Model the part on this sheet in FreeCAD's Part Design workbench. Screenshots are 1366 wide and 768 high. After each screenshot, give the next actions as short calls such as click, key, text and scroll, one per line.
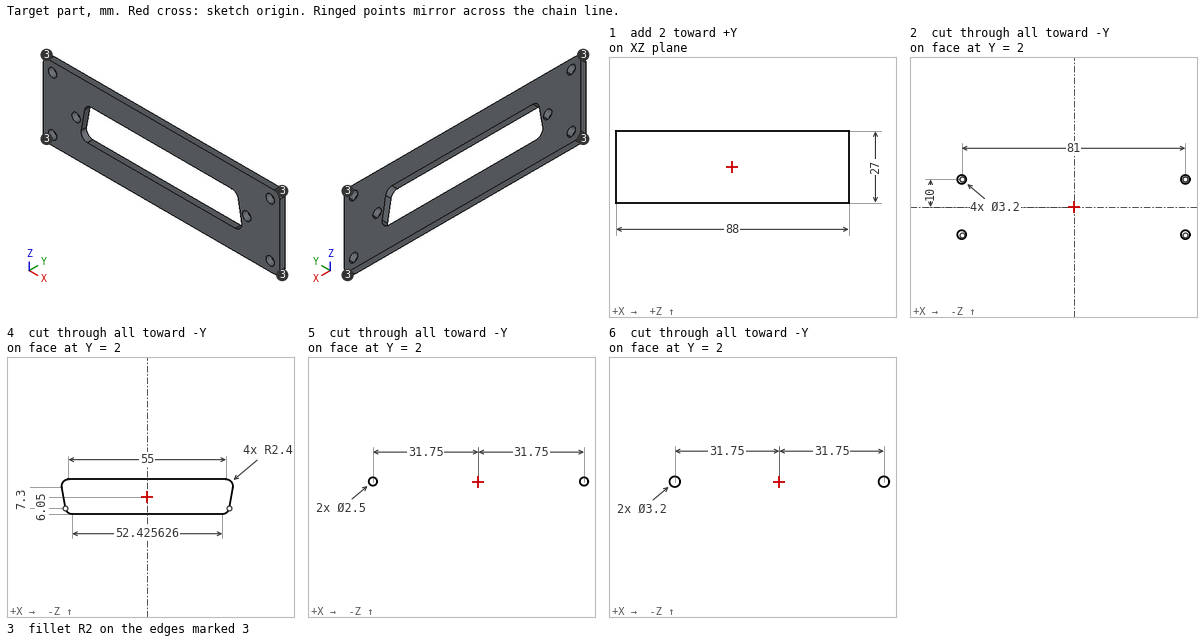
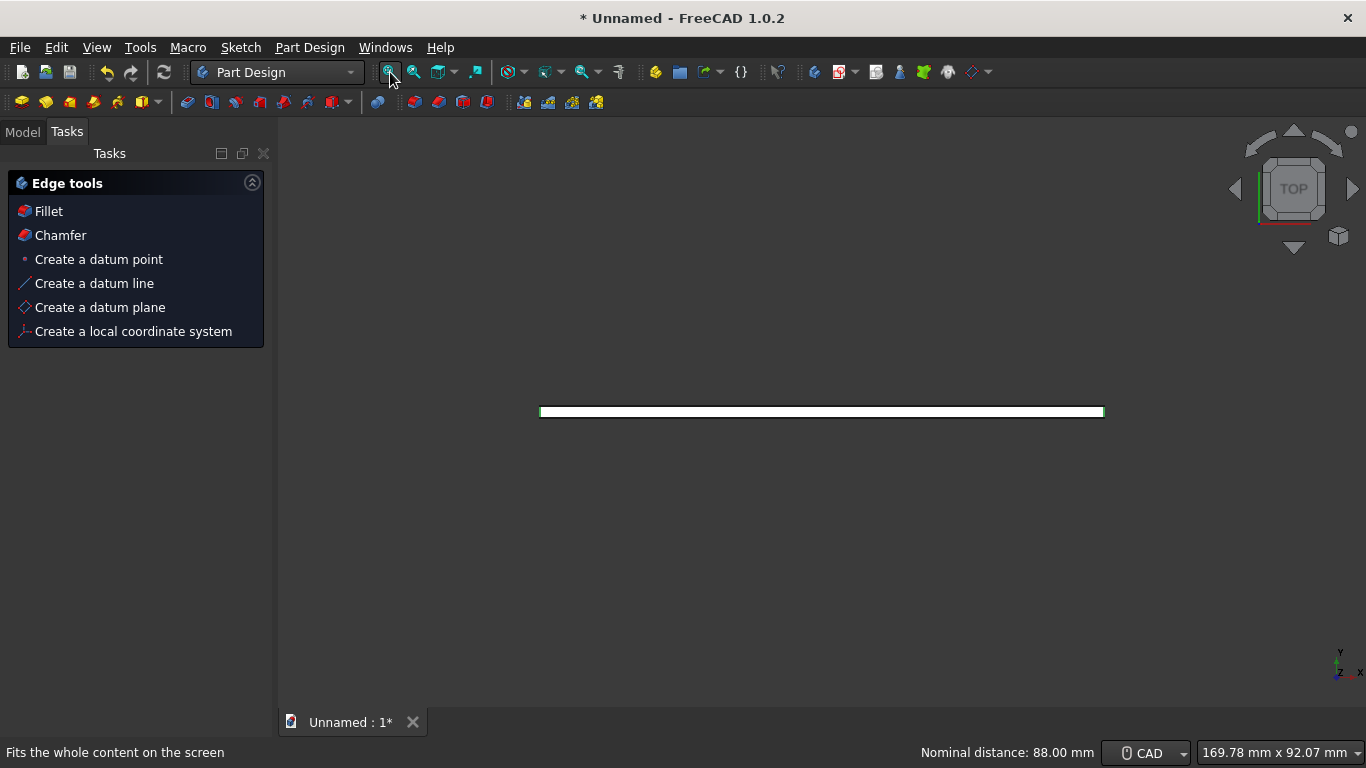
key(1)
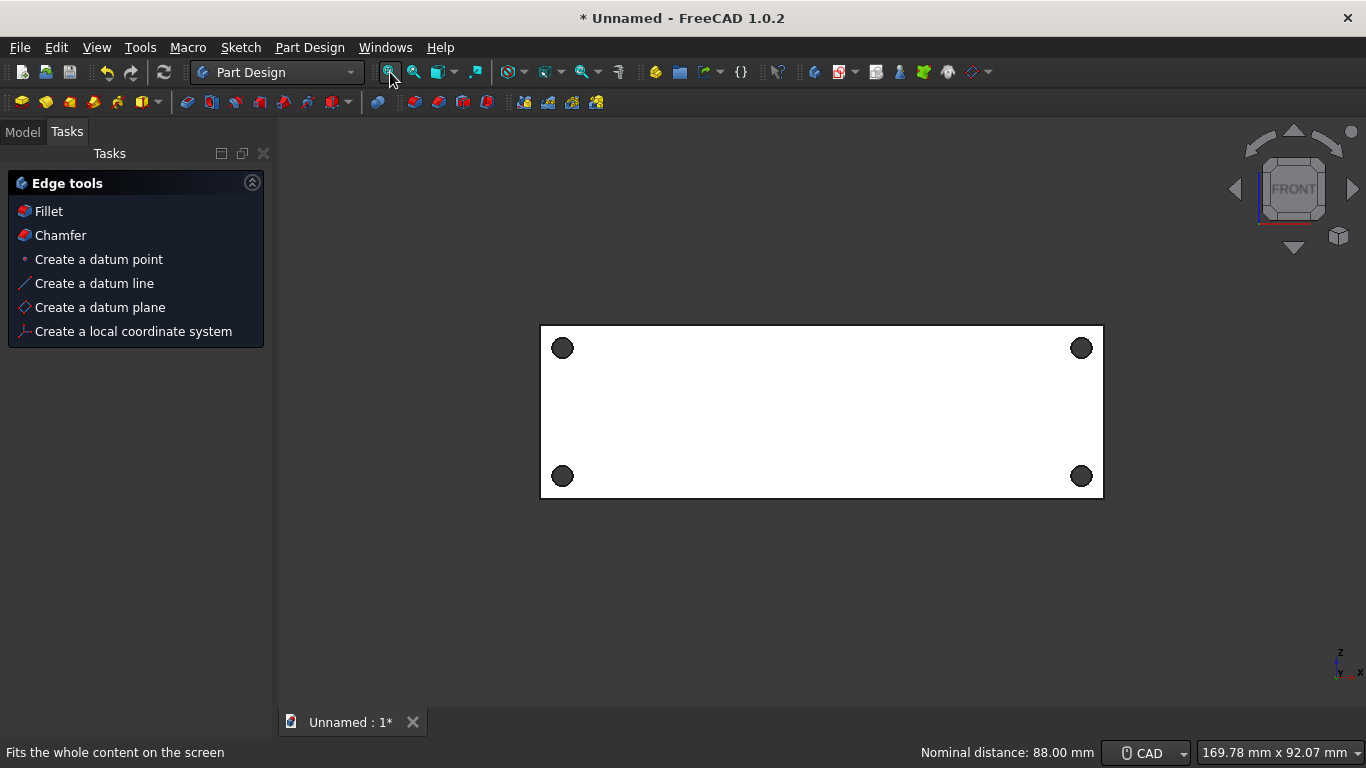
scroll(540, 498, up, 6)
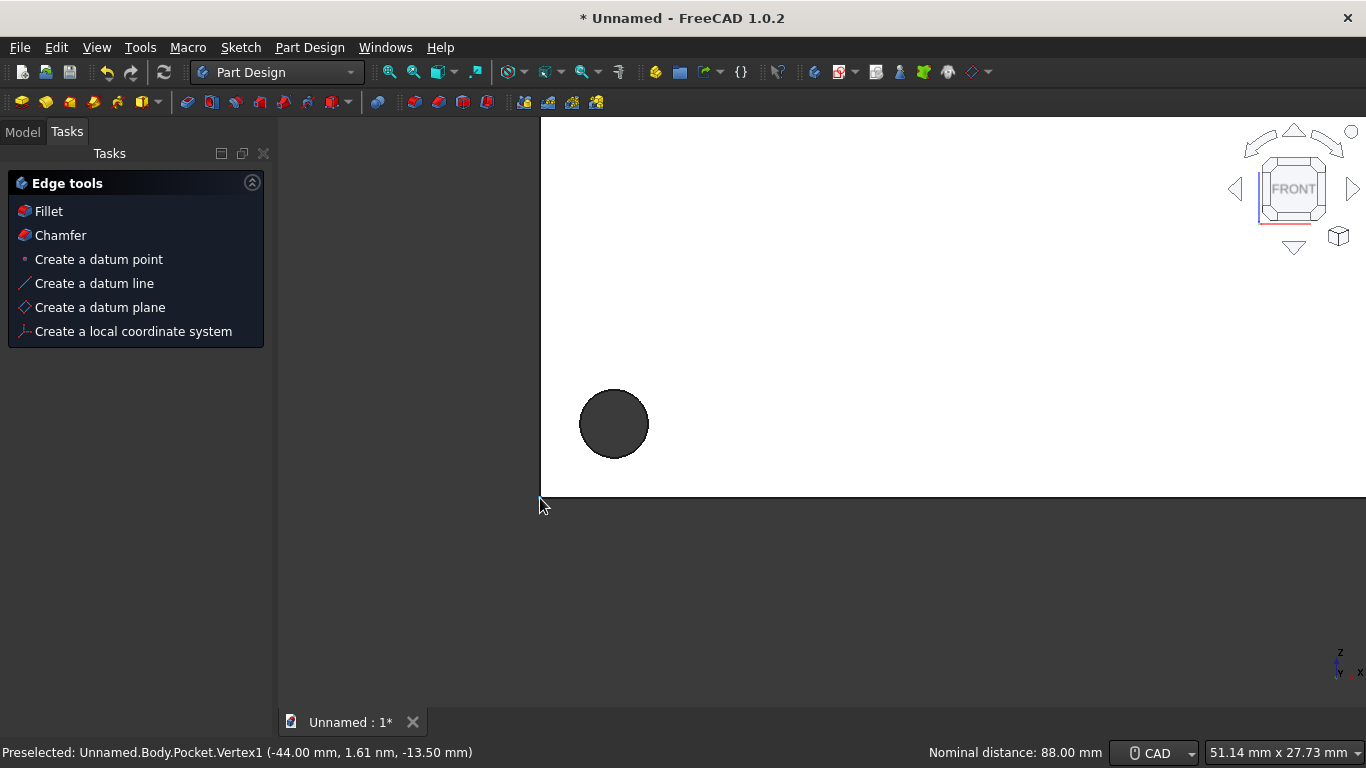
click(390, 72)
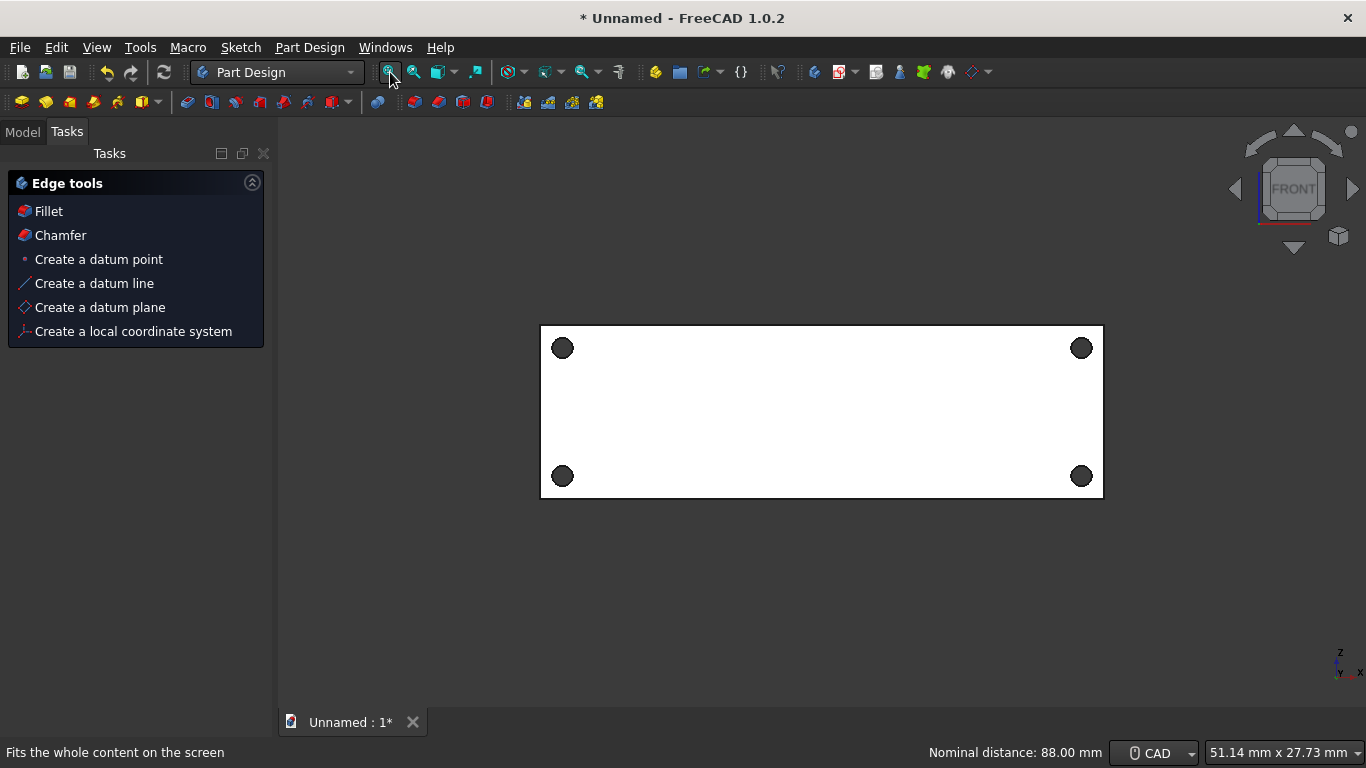
key(3)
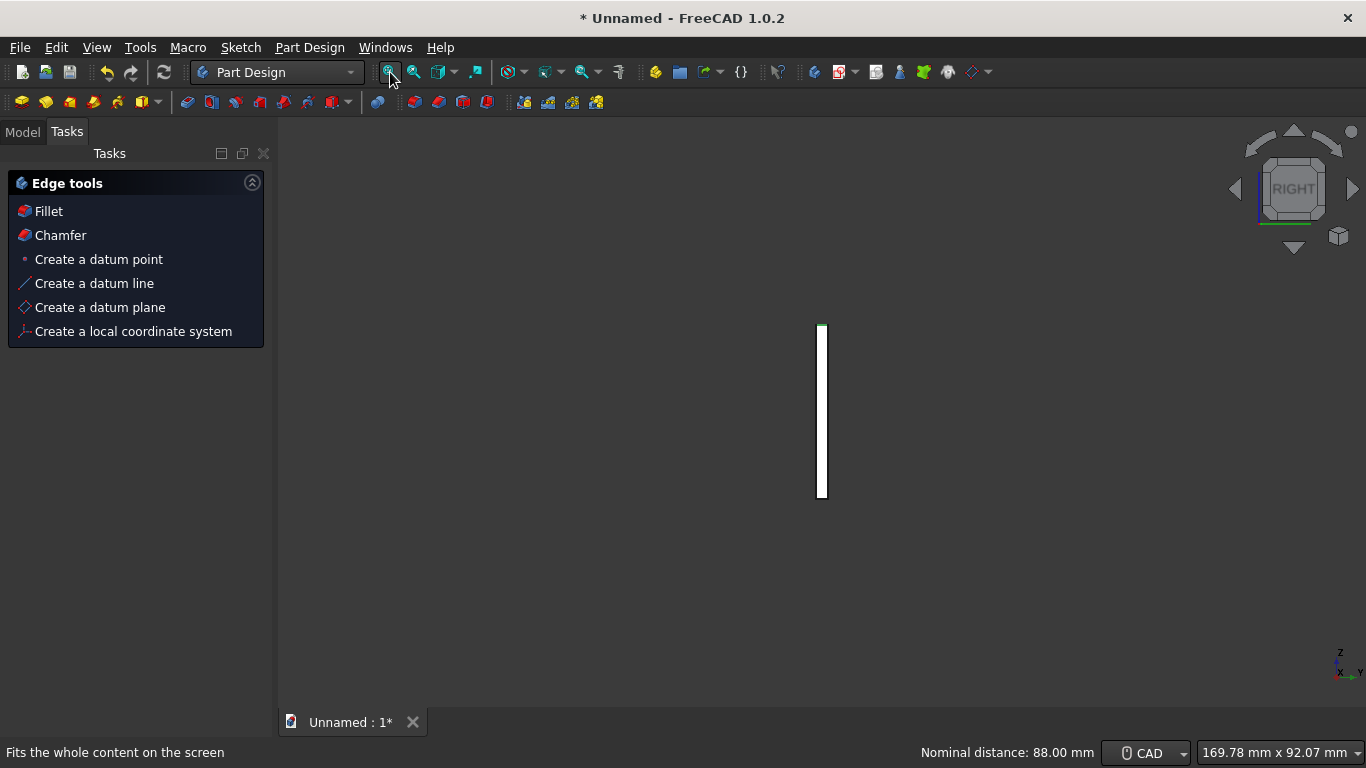
click(390, 72)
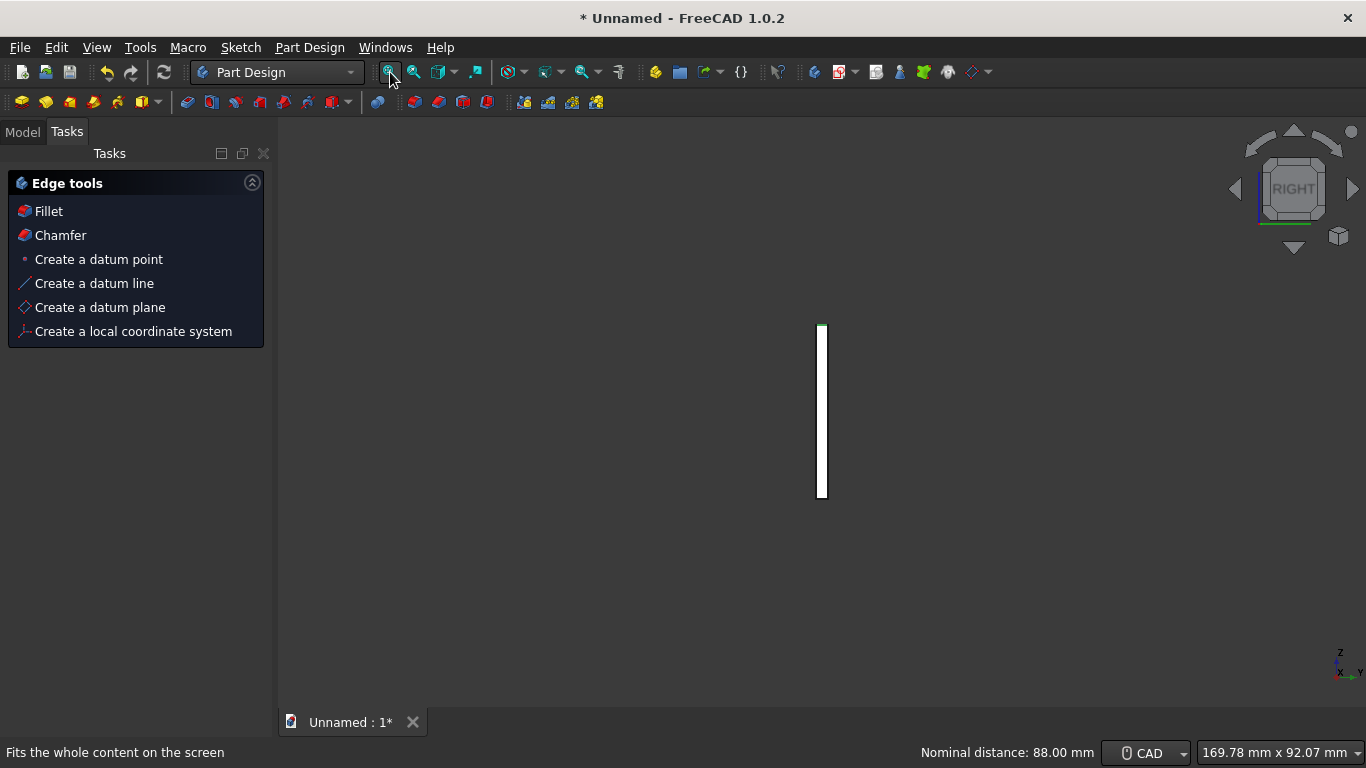
click(822, 498, ctrl)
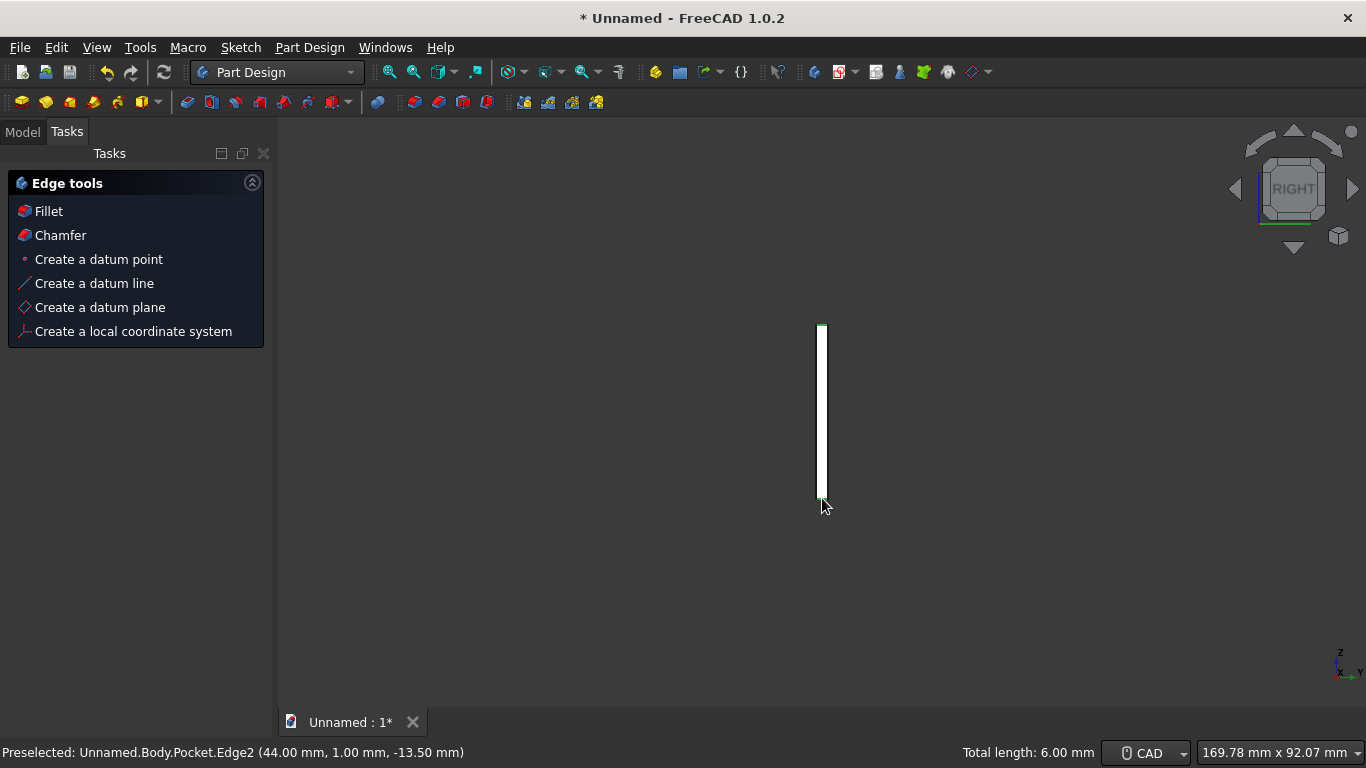
scroll(822, 498, up, 6)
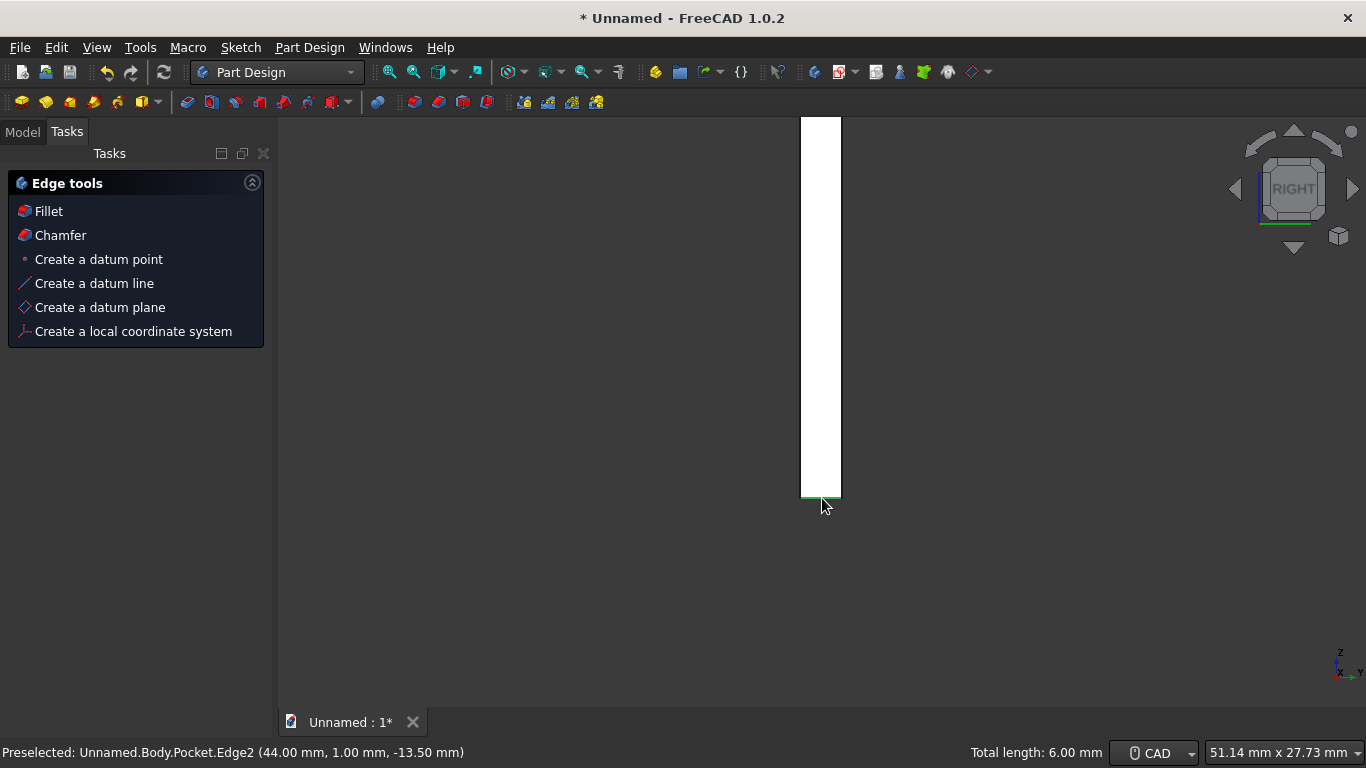
key(v)
key(f)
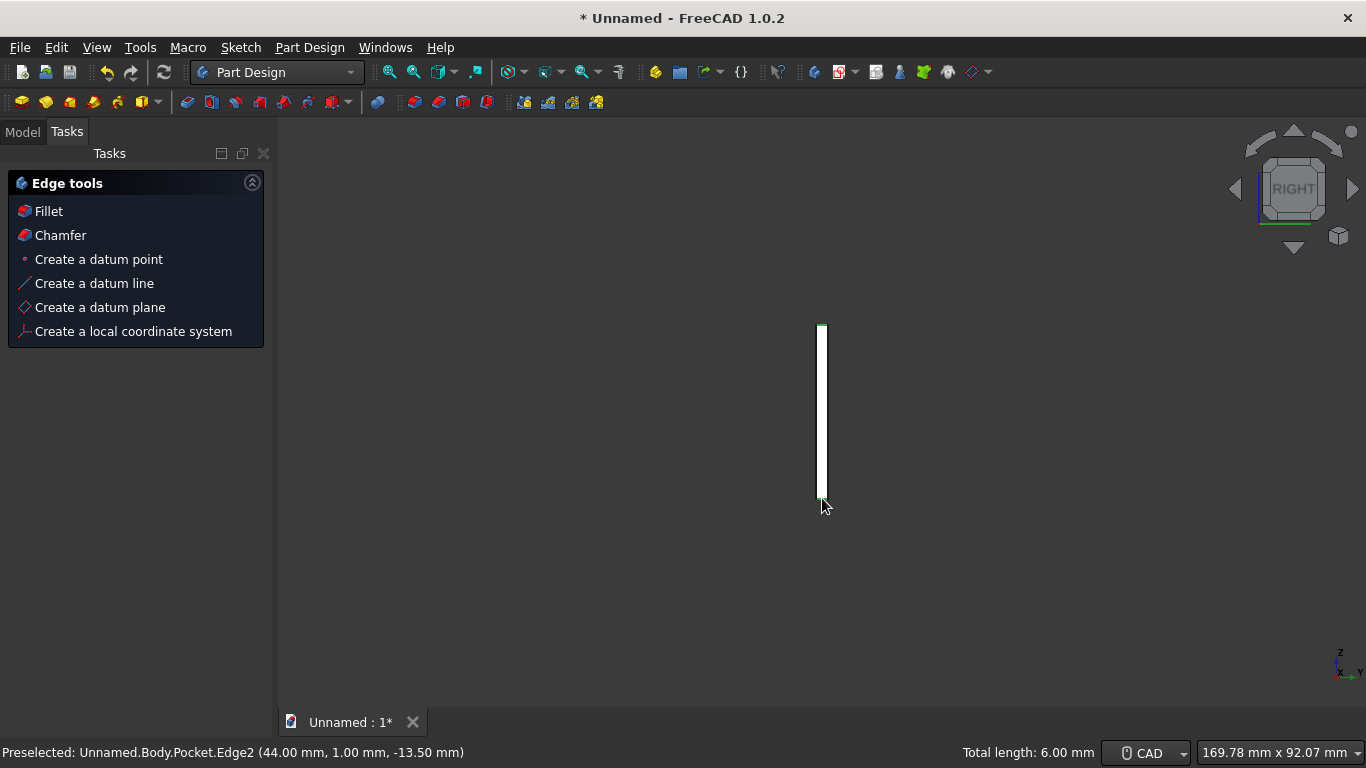
key(5)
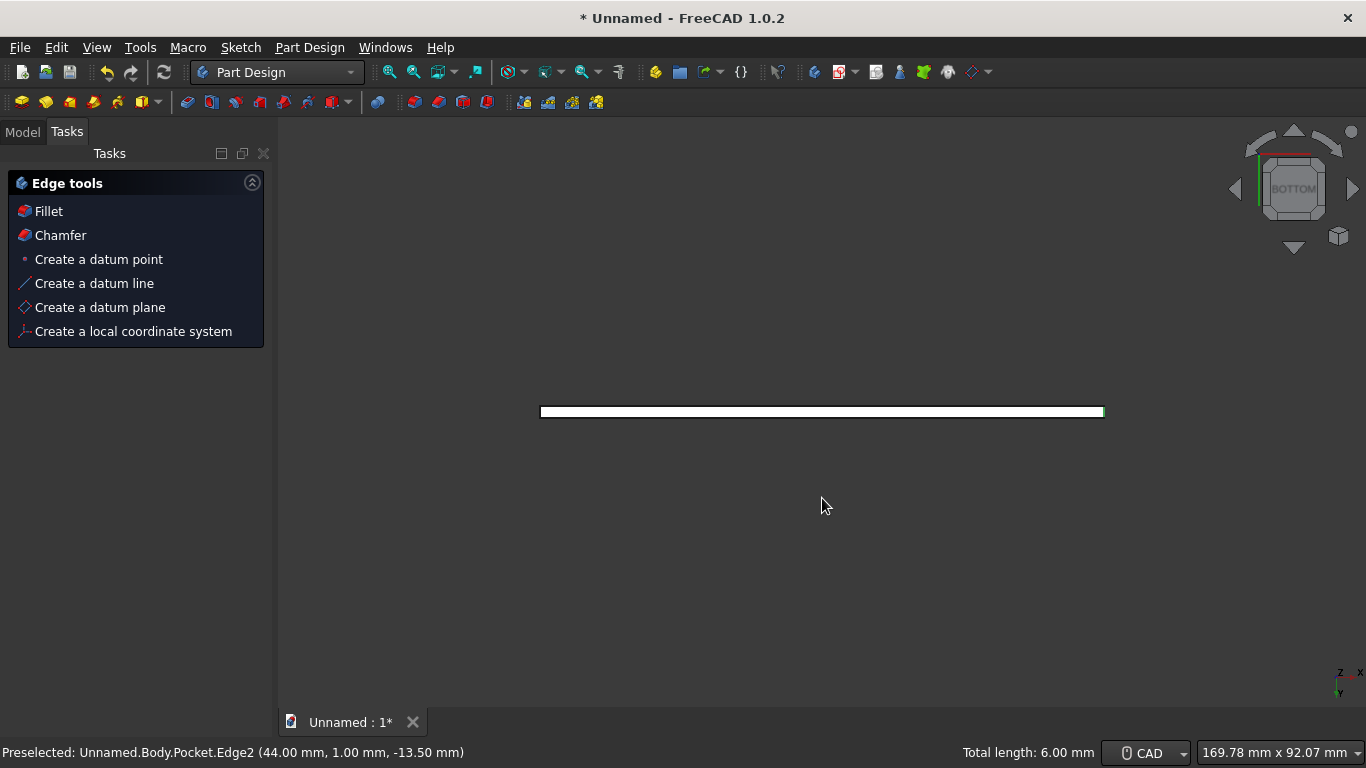
click(540, 411, ctrl)